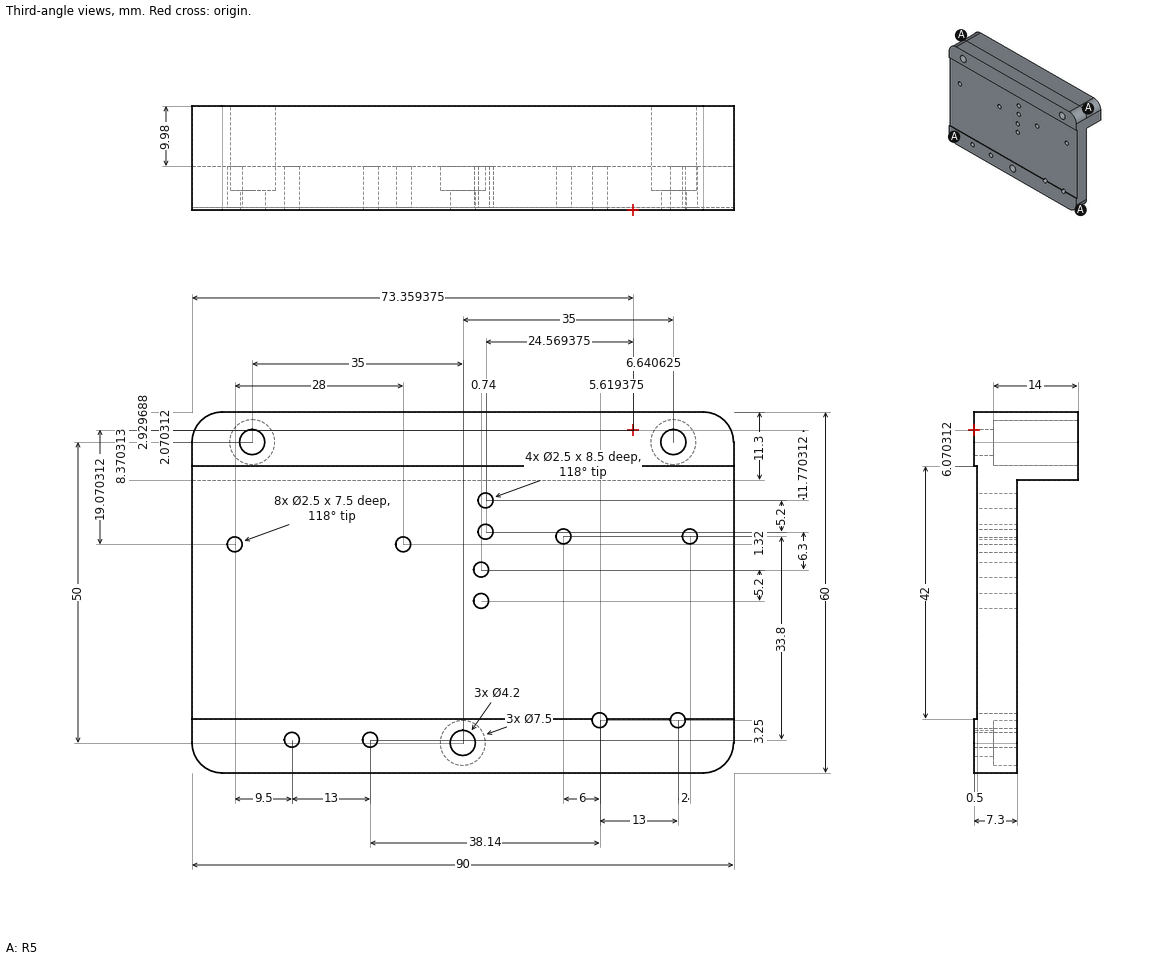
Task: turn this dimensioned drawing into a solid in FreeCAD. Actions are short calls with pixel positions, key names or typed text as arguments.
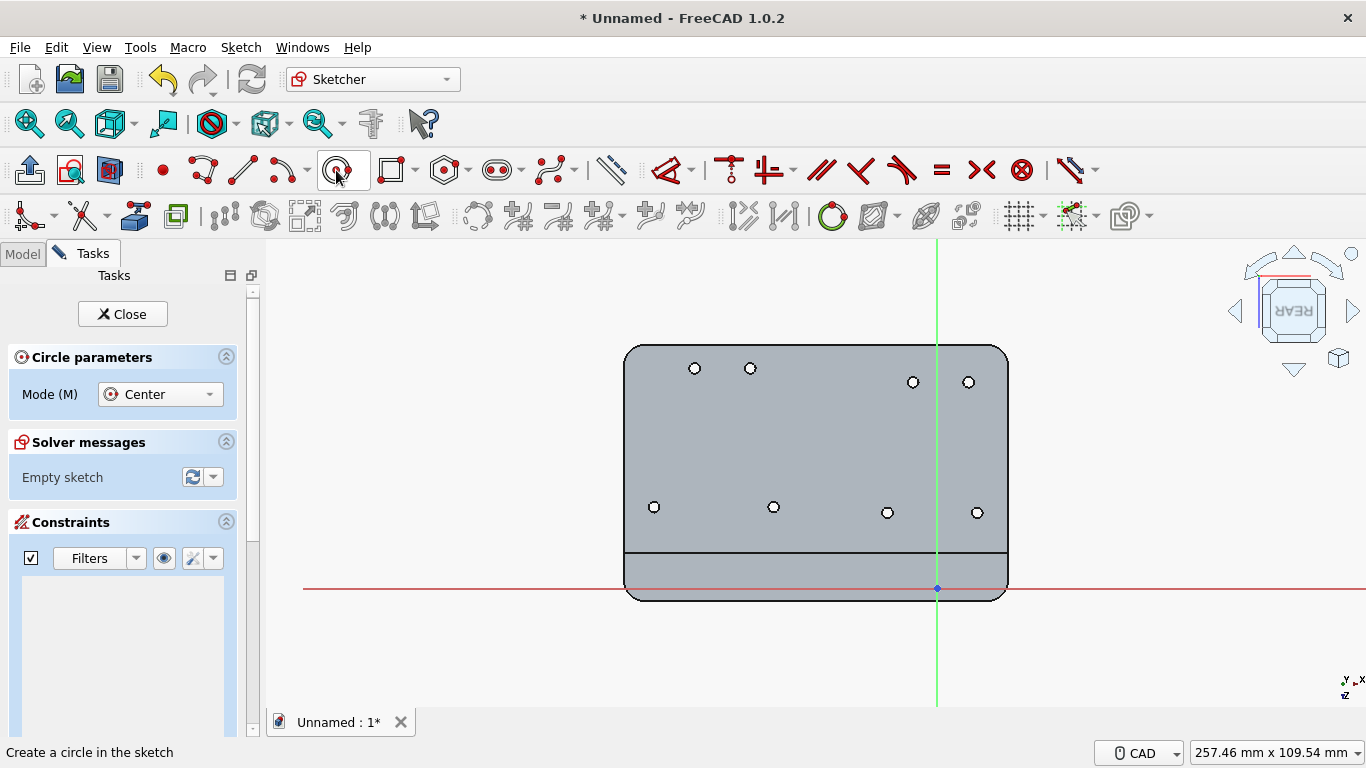
scroll(816, 366, up, 2)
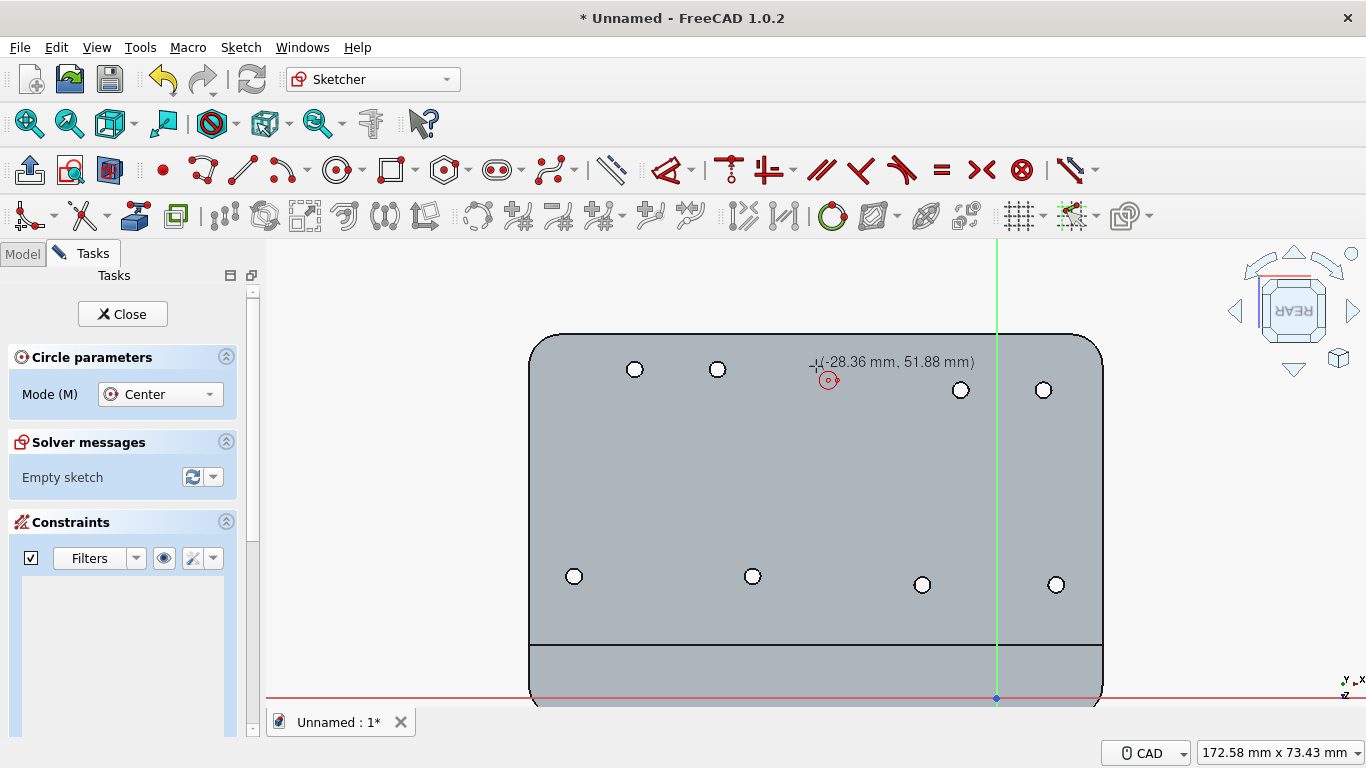
click(816, 366)
move(833, 349)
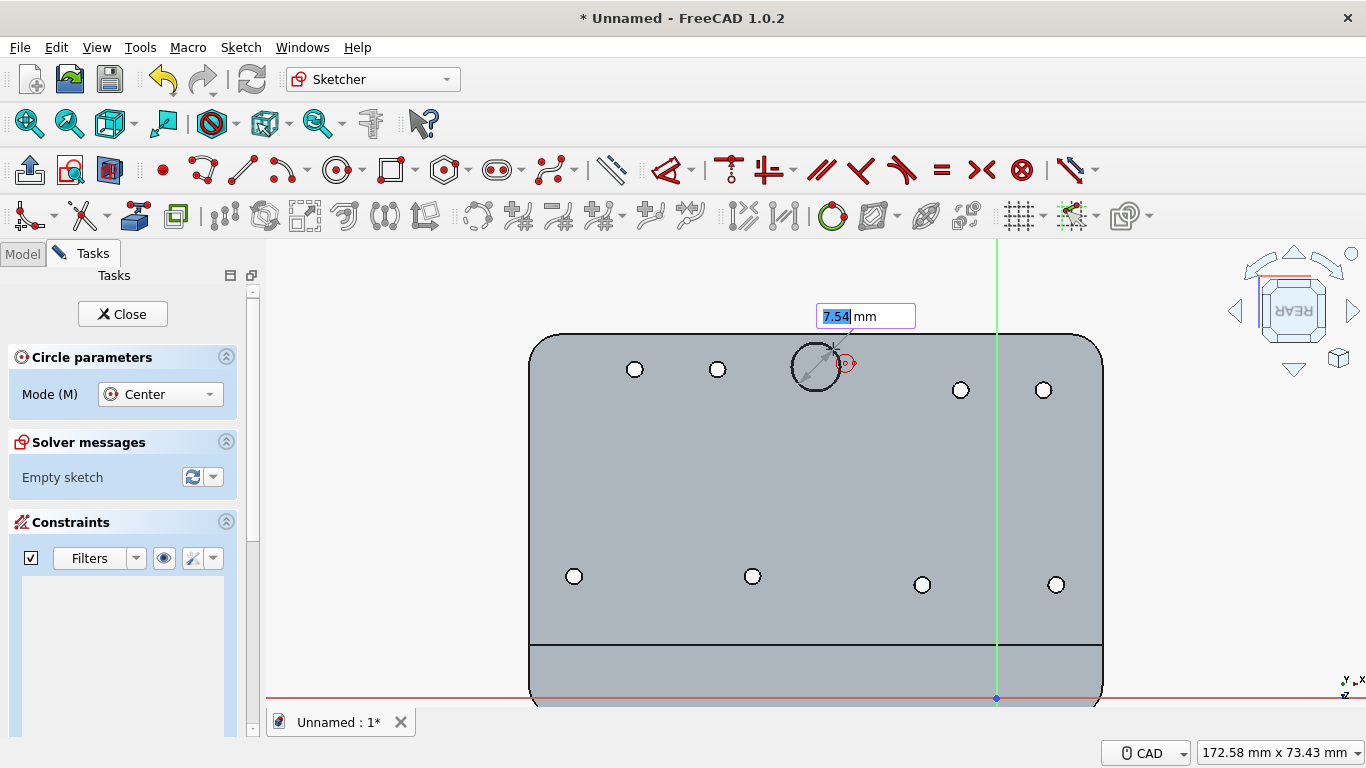
text(7.5)
key(Return)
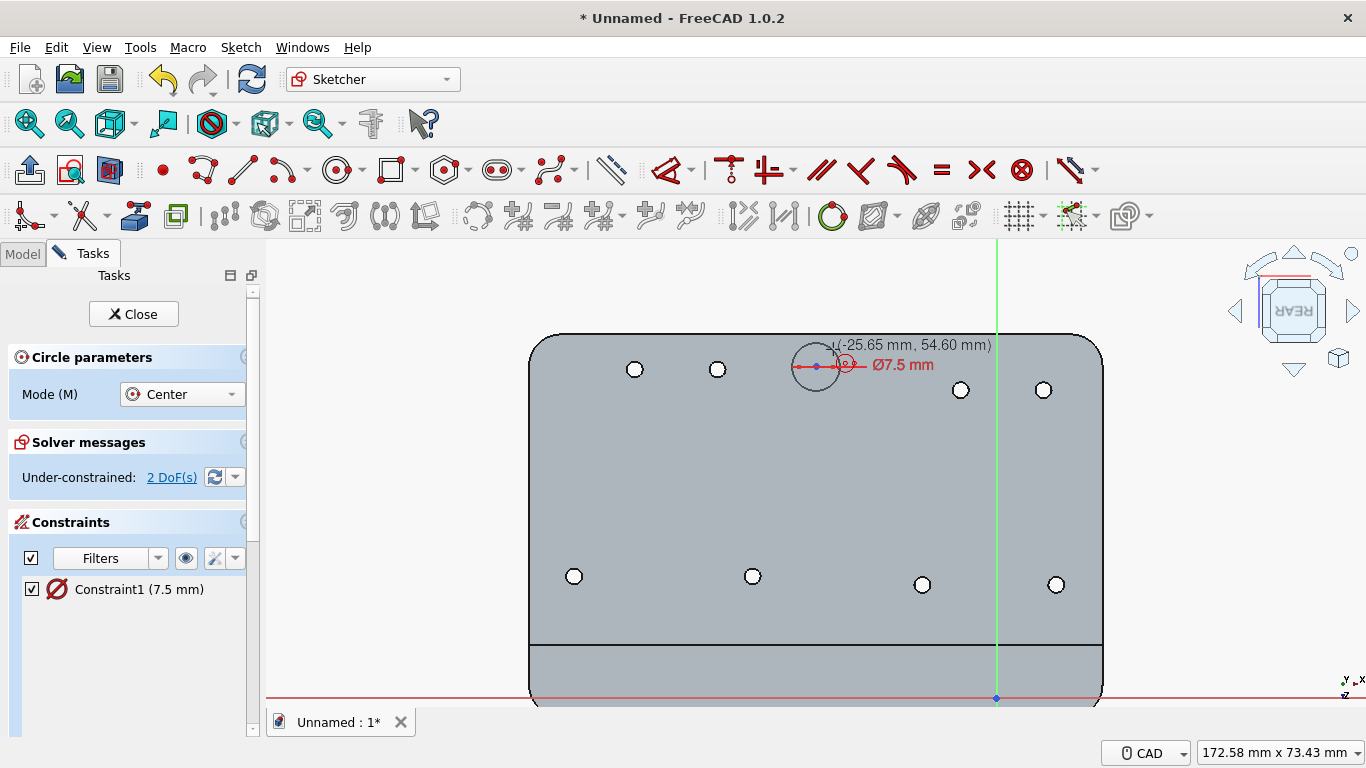
scroll(439, 267, down, 1)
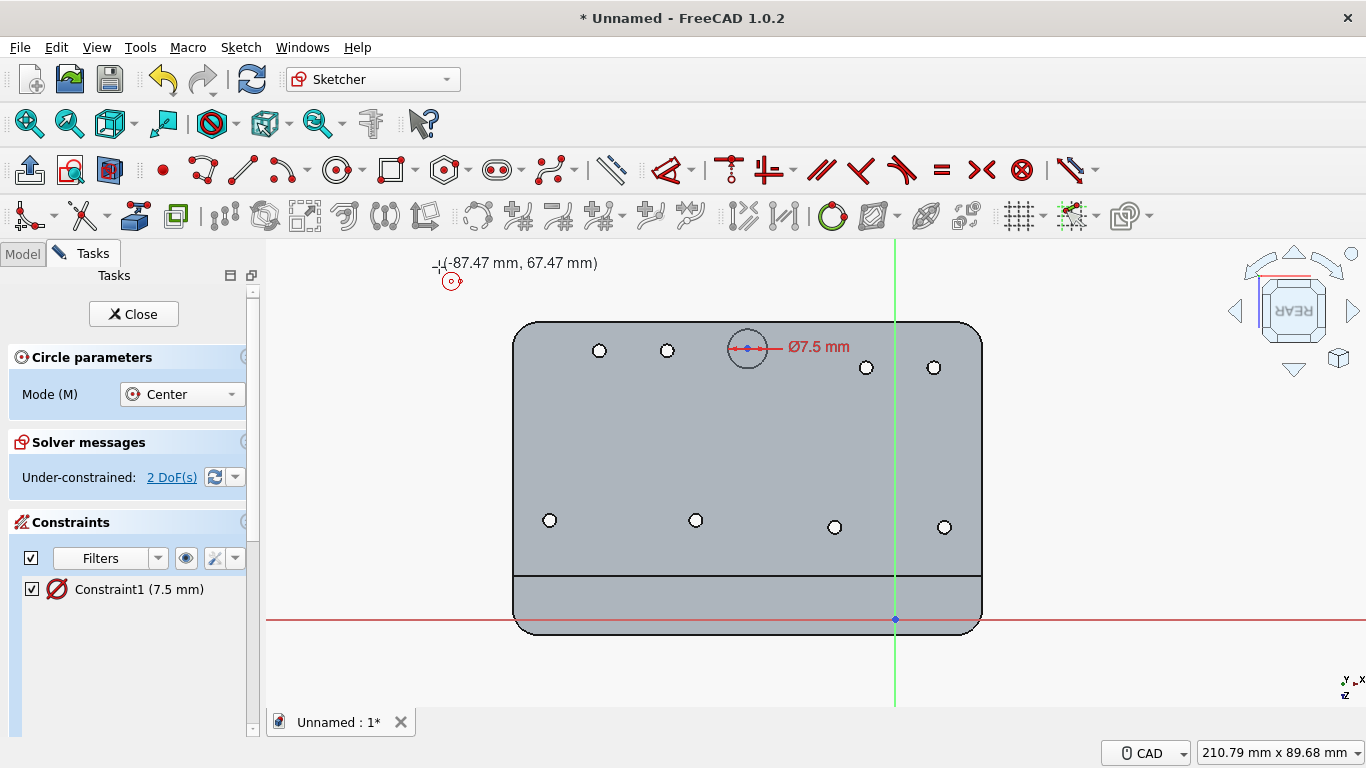
scroll(565, 609, up, 2)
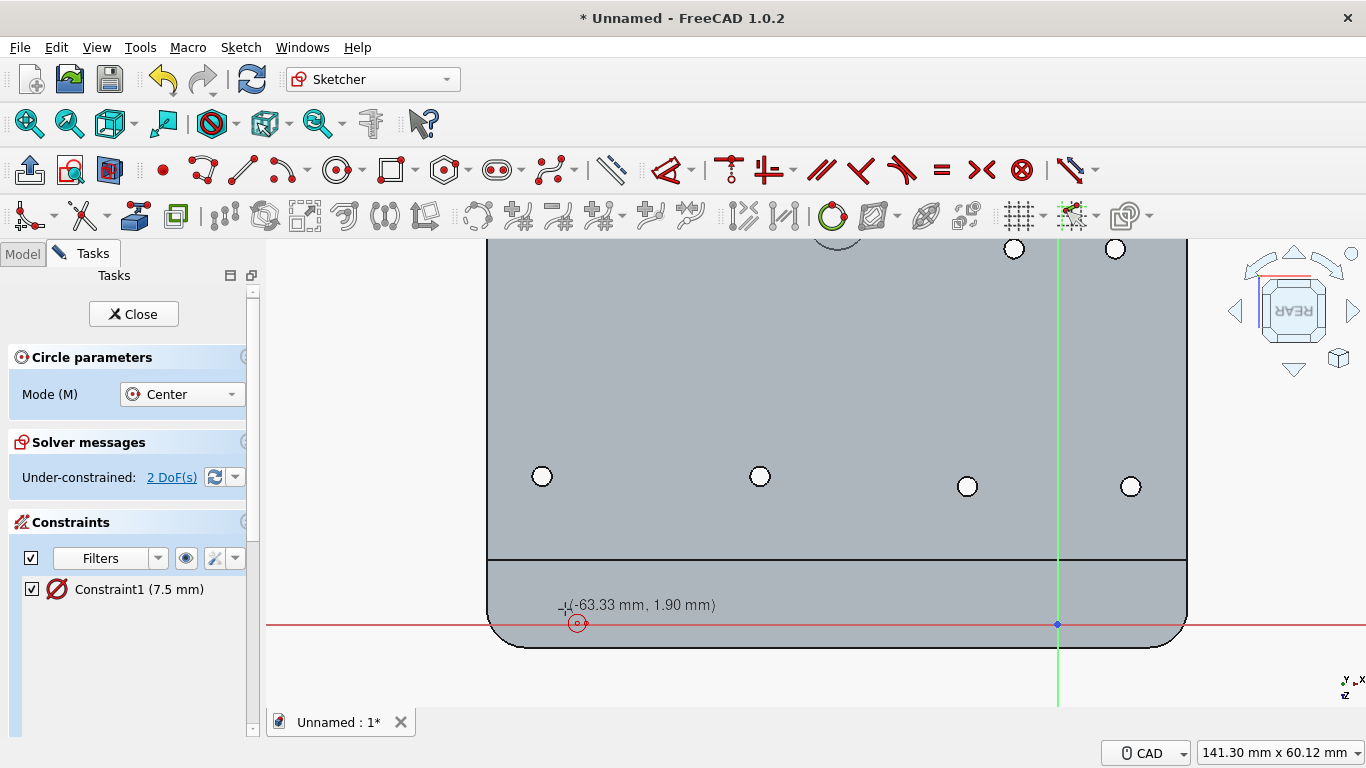
click(565, 609)
move(585, 588)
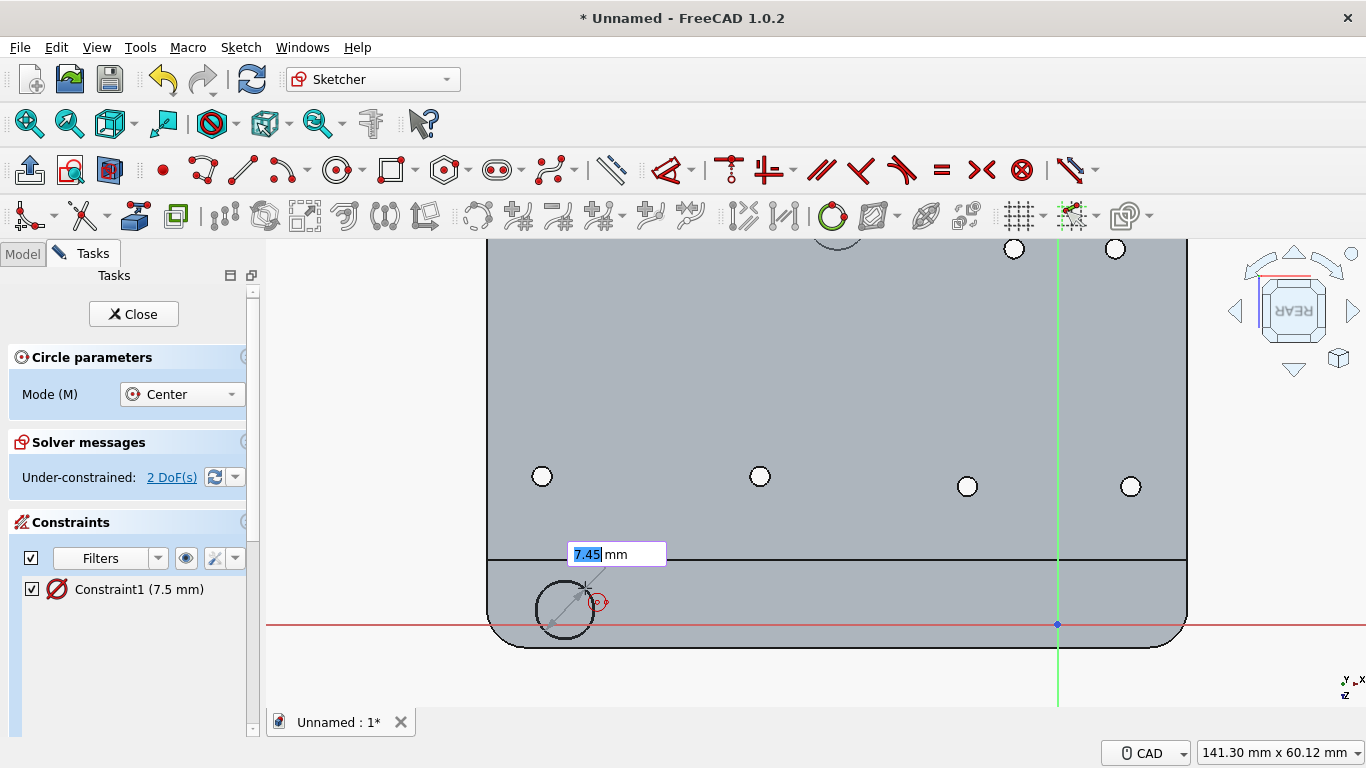
text(7.5)
key(Return)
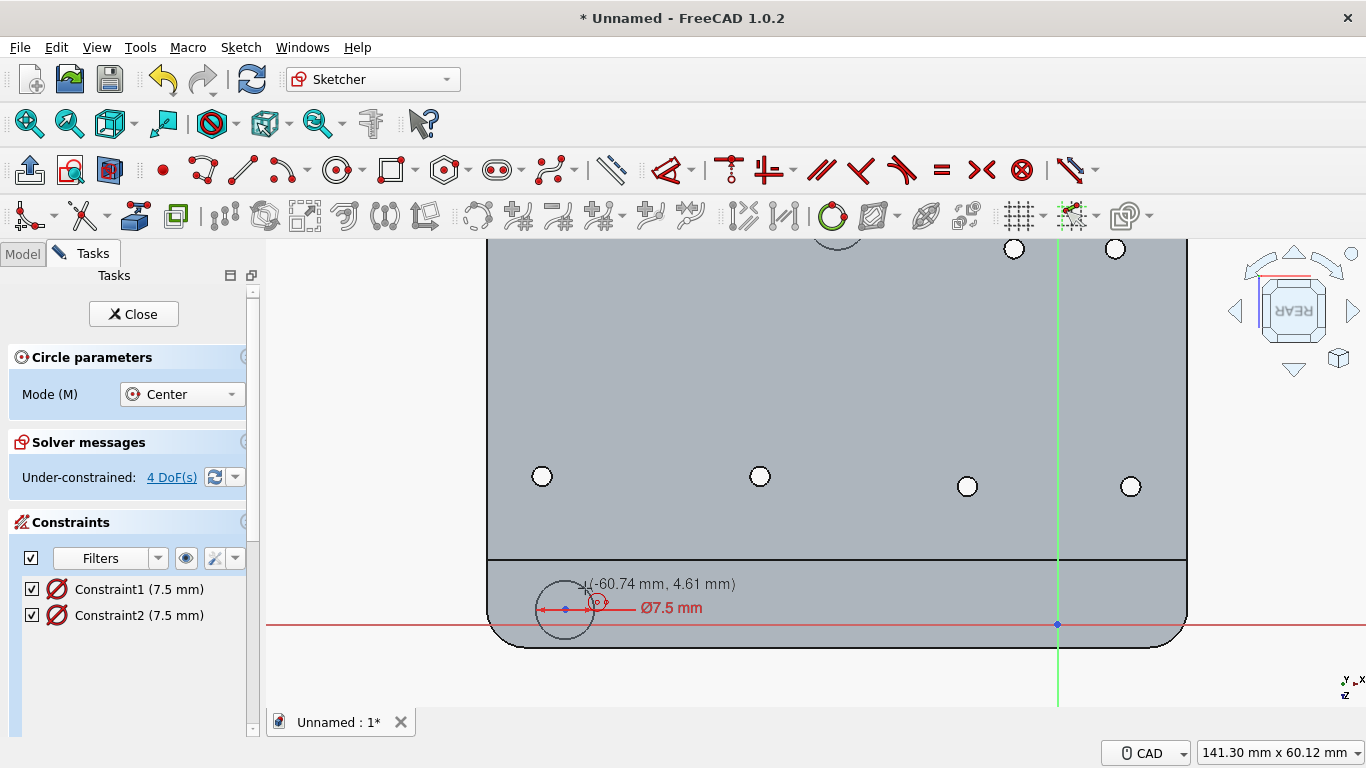
click(1110, 609)
move(1130, 588)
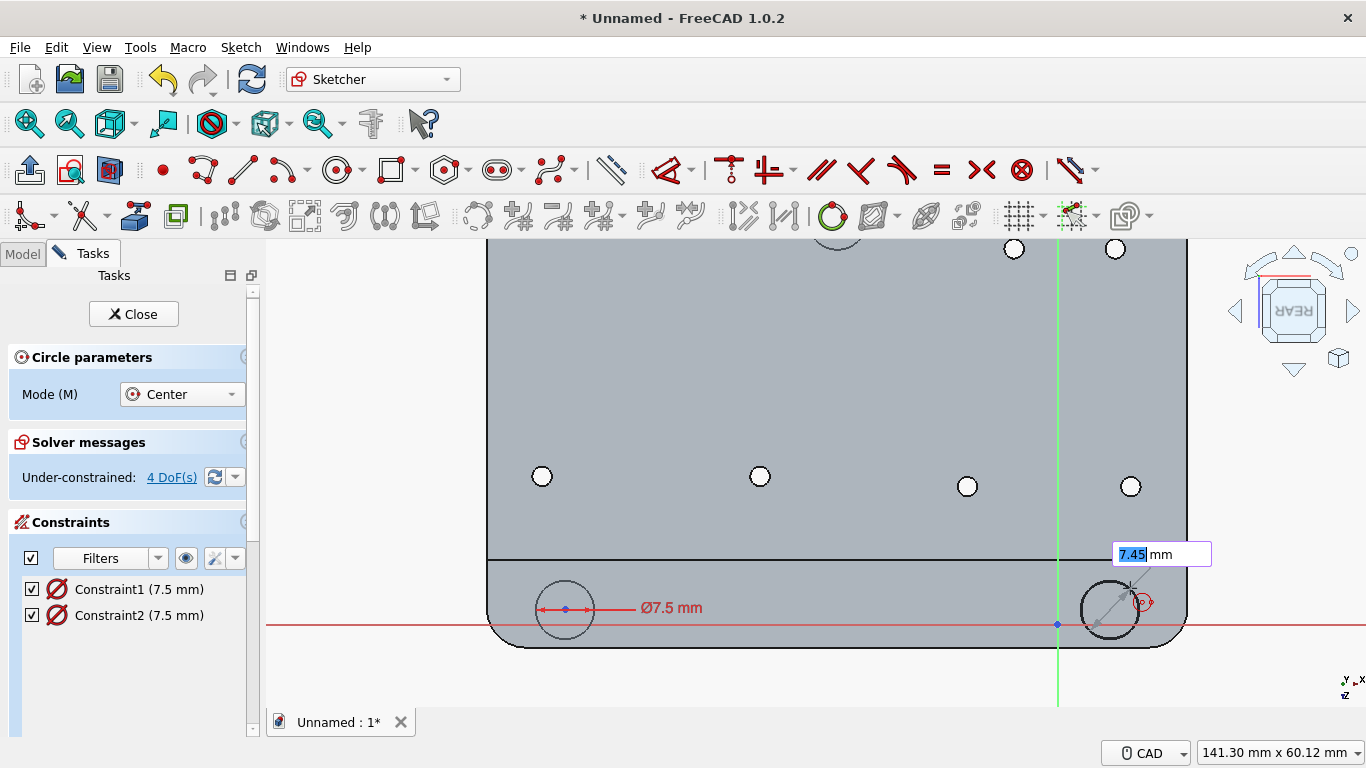
text(7.5)
key(Return)
key(Escape)